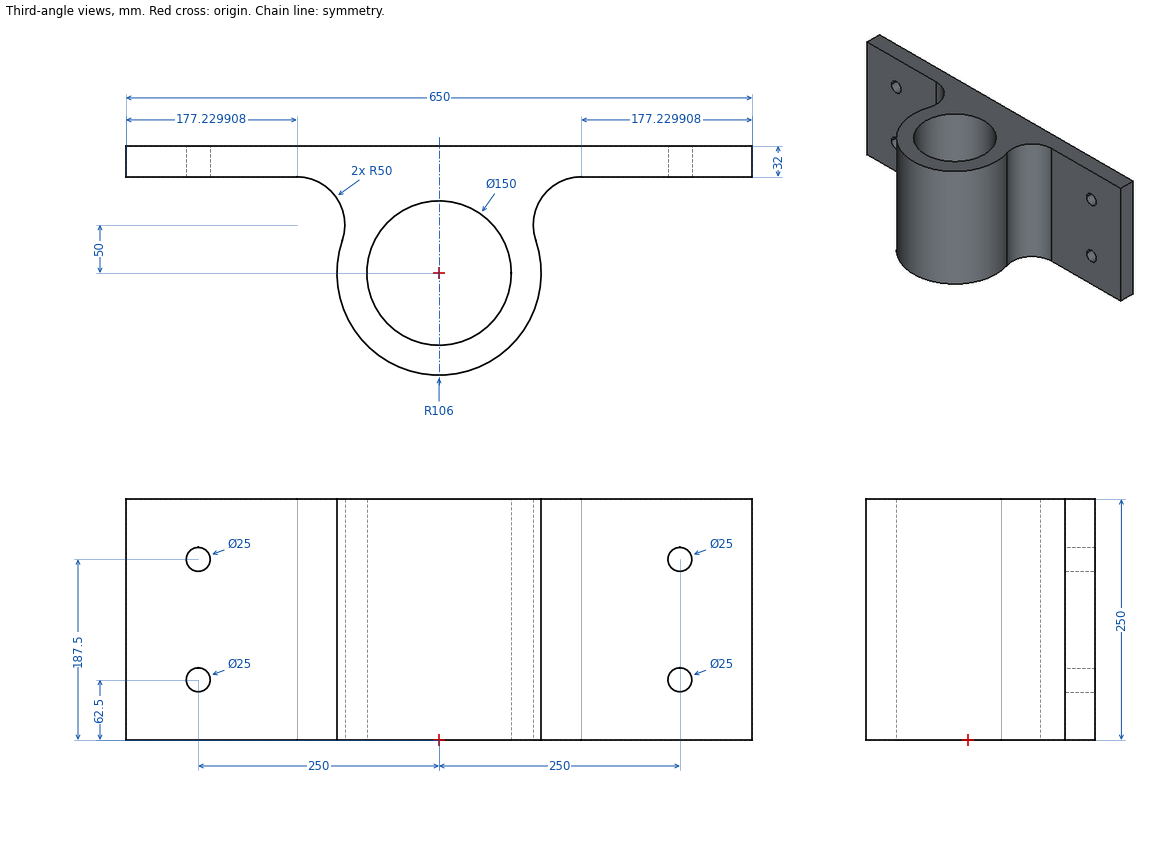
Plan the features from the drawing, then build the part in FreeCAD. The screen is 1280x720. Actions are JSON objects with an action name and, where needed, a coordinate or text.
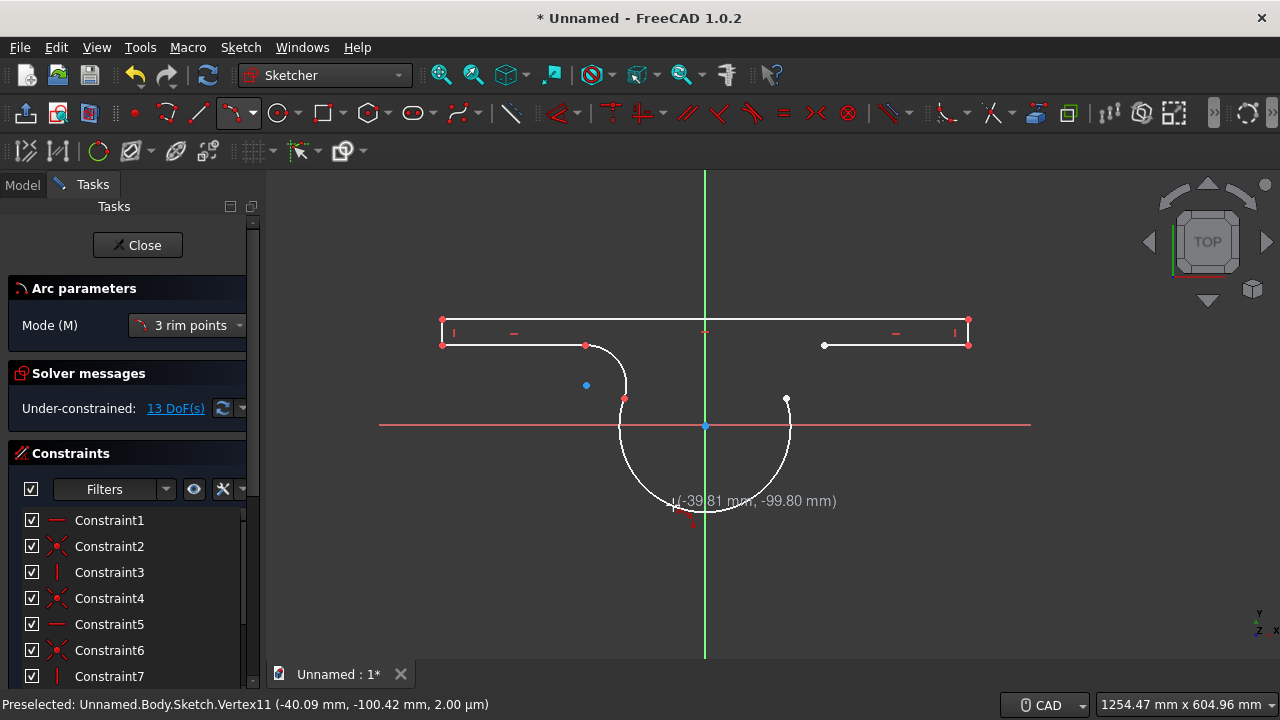
{"action": "left_click", "coordinate": [786, 399]}
{"action": "left_click", "coordinate": [825, 345]}
{"action": "left_click", "coordinate": [792, 361]}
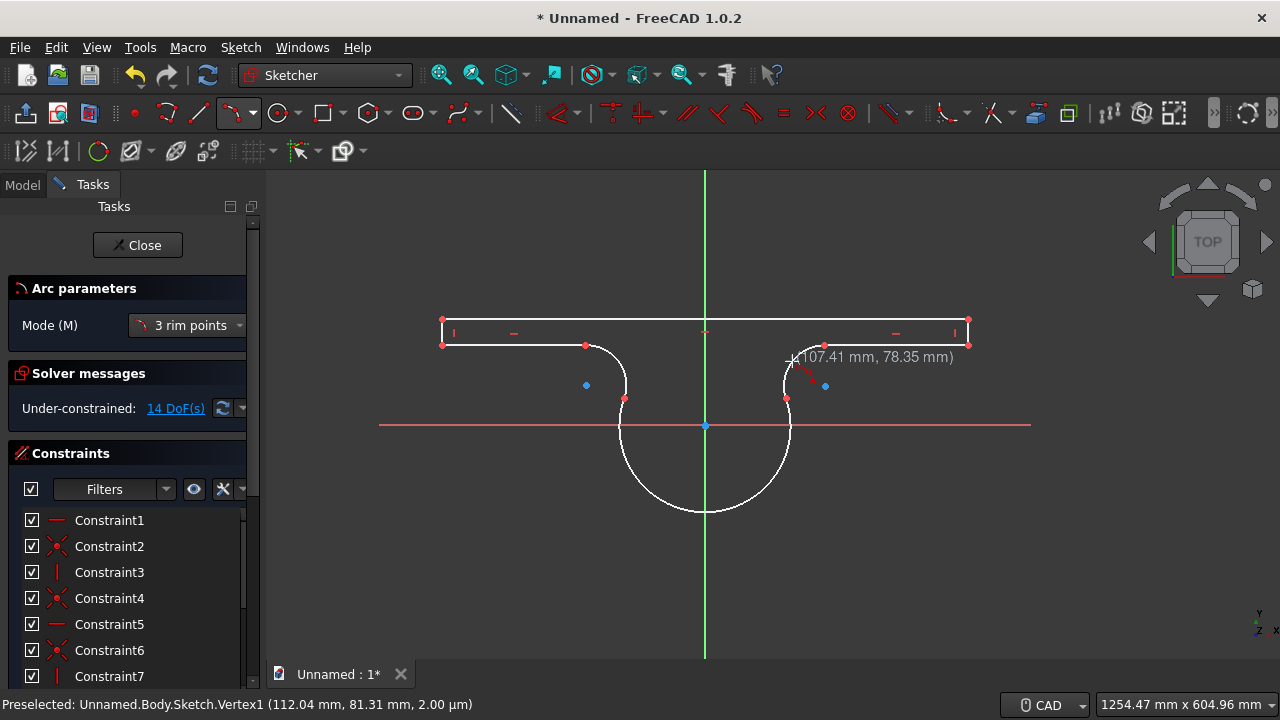
{"action": "left_click", "coordinate": [278, 114]}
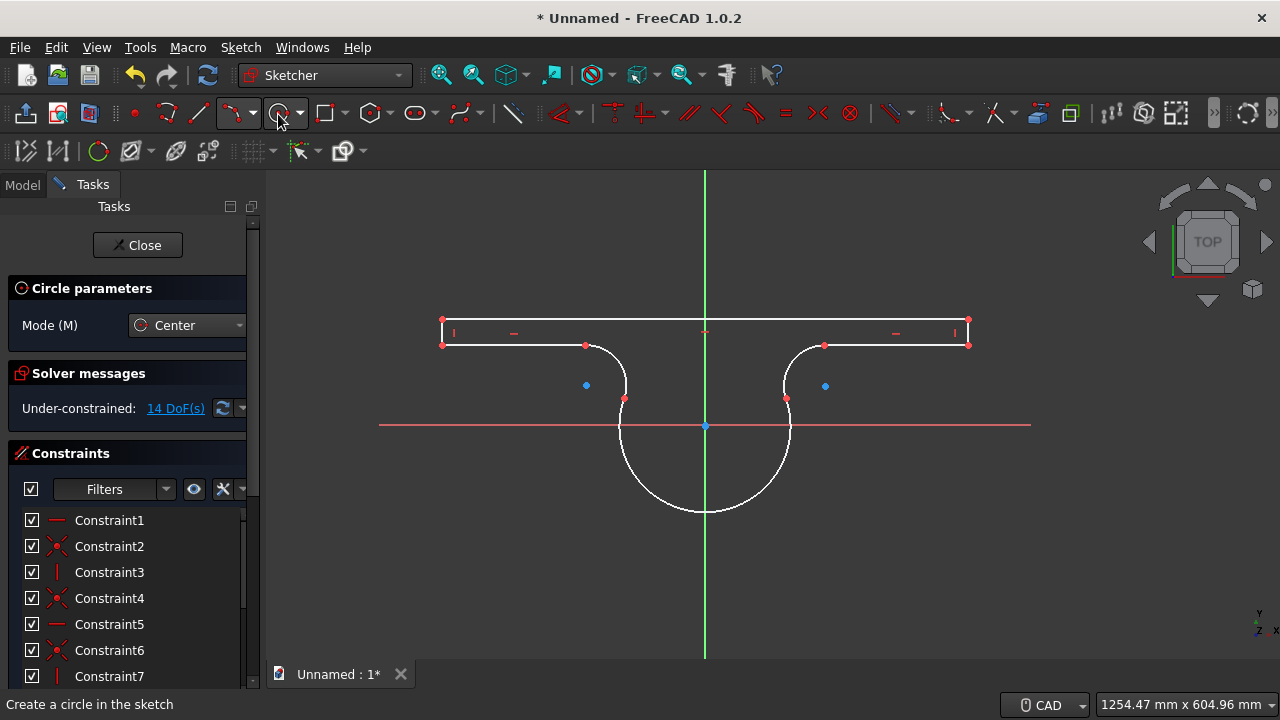
{"action": "left_click", "coordinate": [705, 425]}
{"action": "mouse_move", "coordinate": [748, 382]}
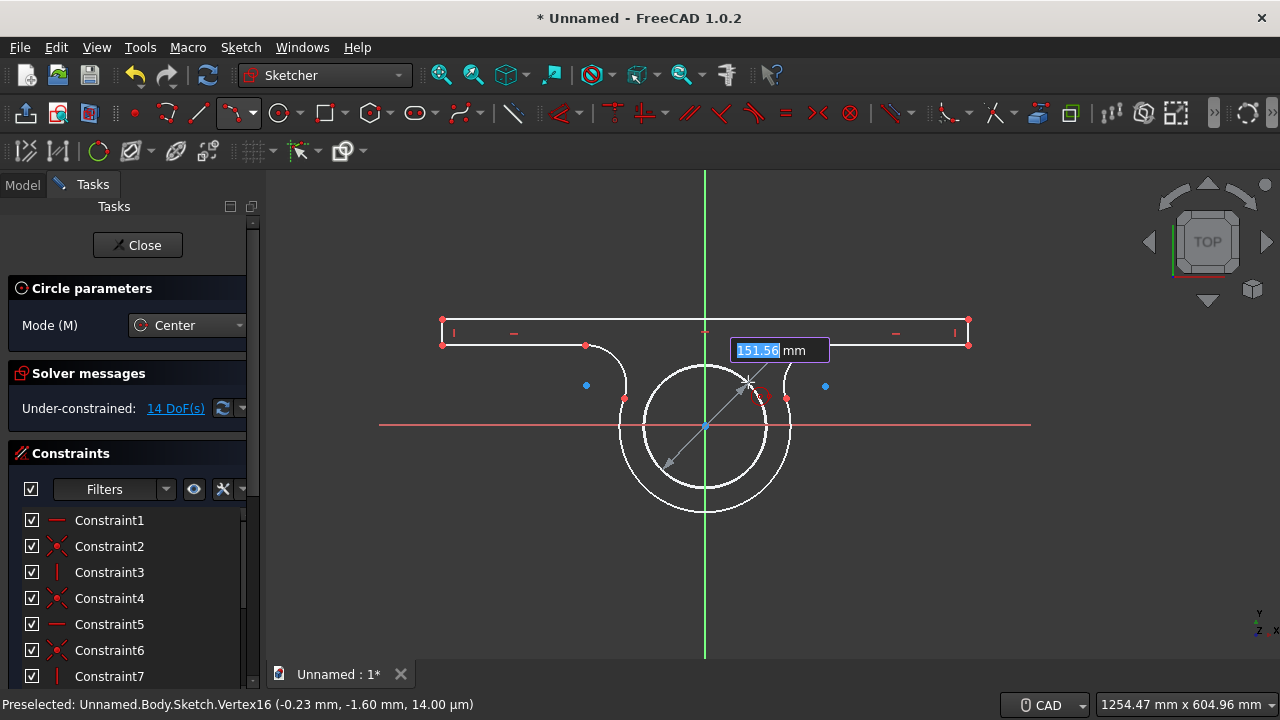
{"action": "type", "text": "150"}
{"action": "key", "text": "Return"}
{"action": "key", "text": "Escape"}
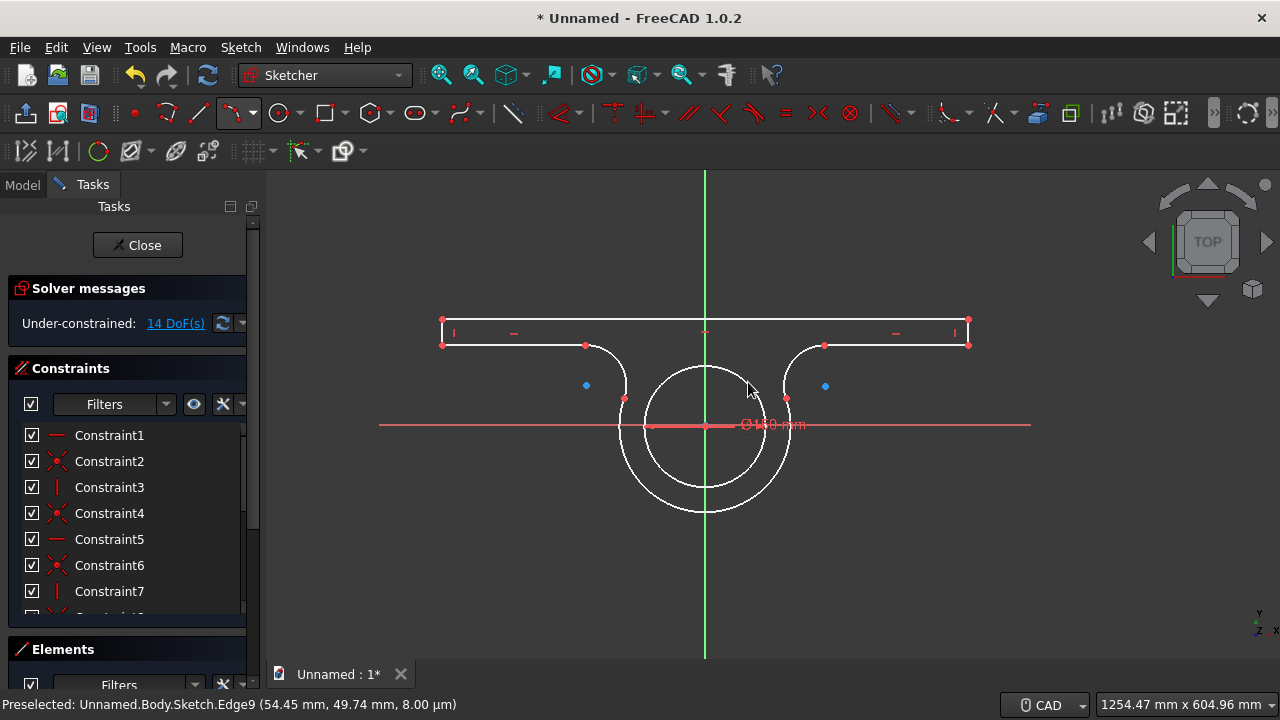
{"action": "left_click", "coordinate": [625, 376]}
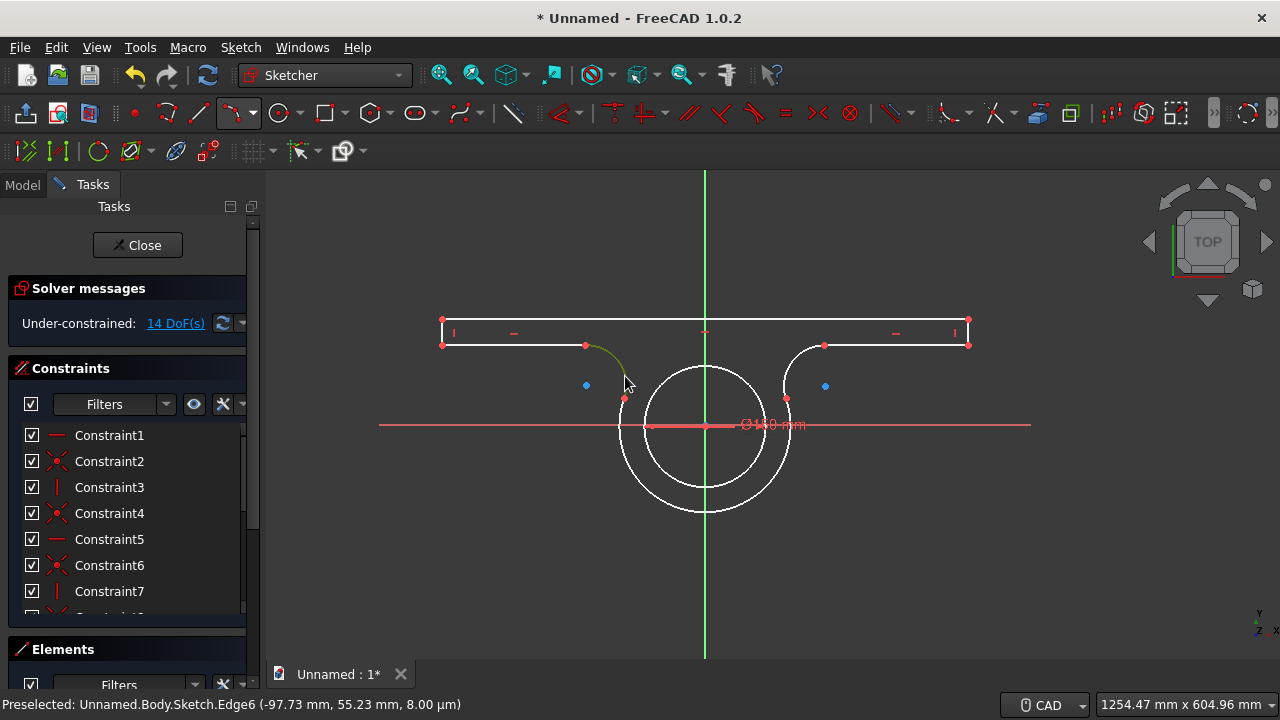
{"action": "left_click", "coordinate": [646, 489]}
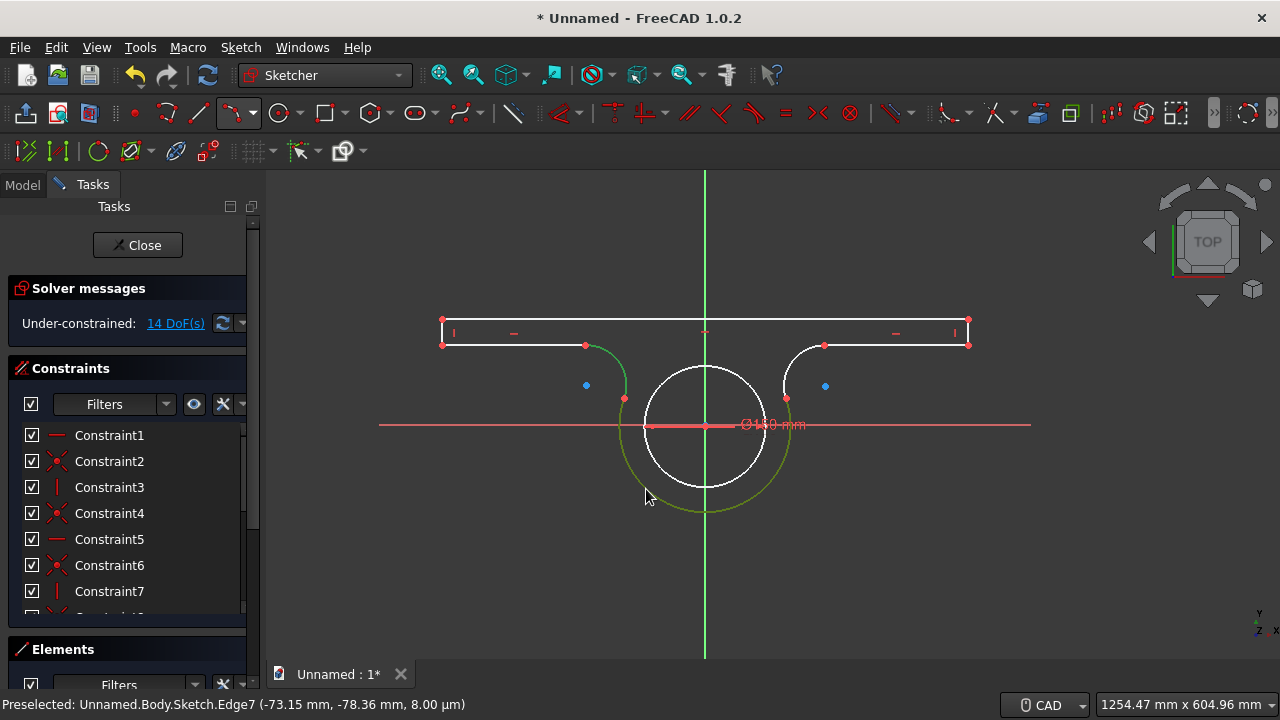
{"action": "left_click", "coordinate": [754, 114]}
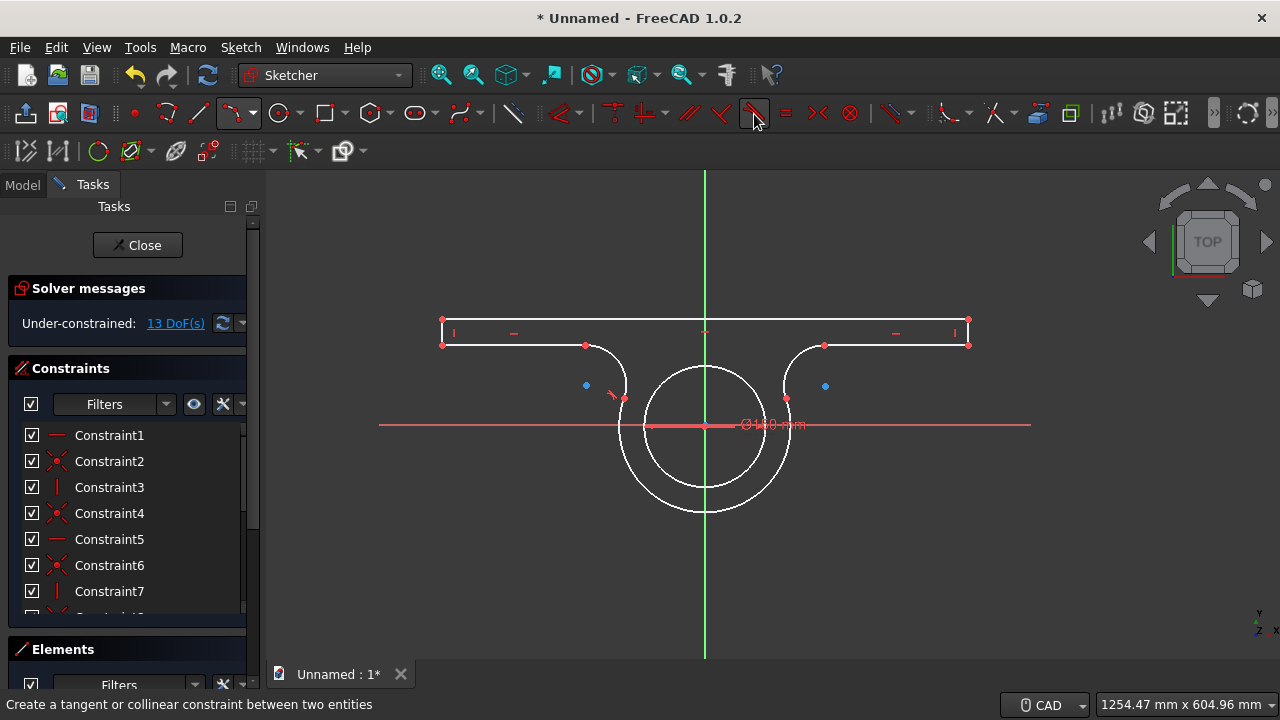
{"action": "left_click", "coordinate": [645, 488]}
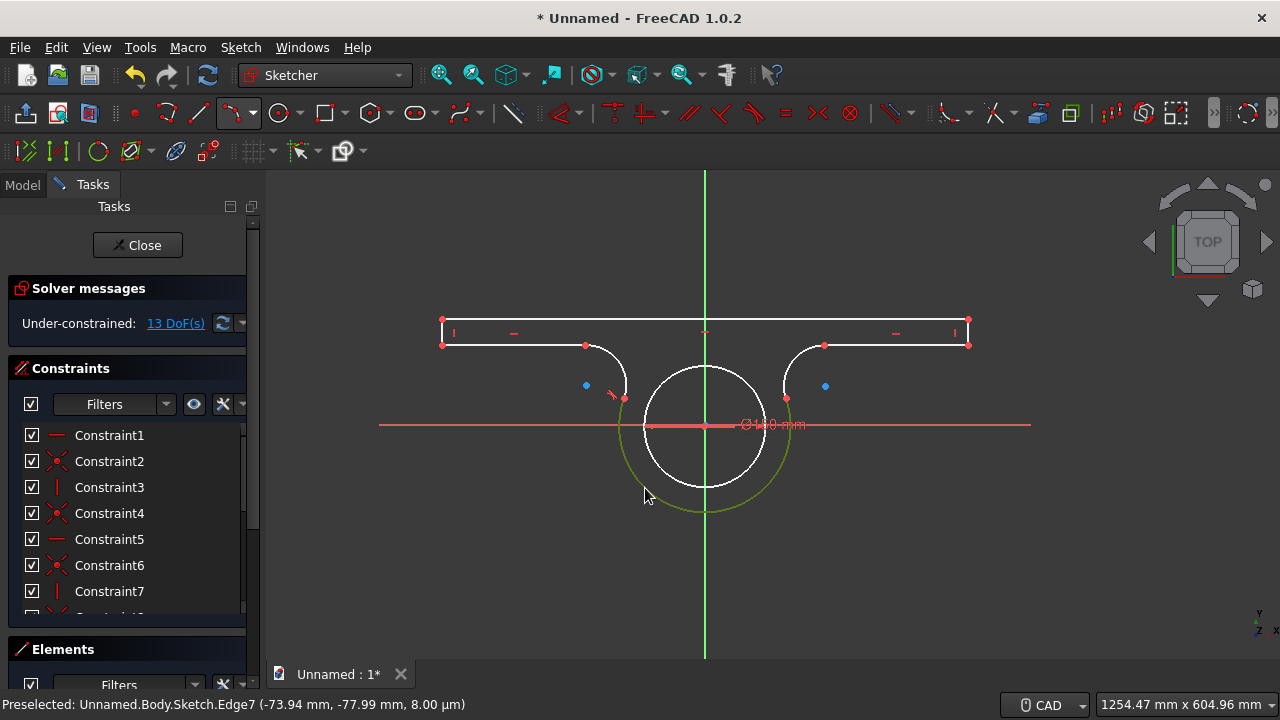
{"action": "left_click", "coordinate": [803, 352]}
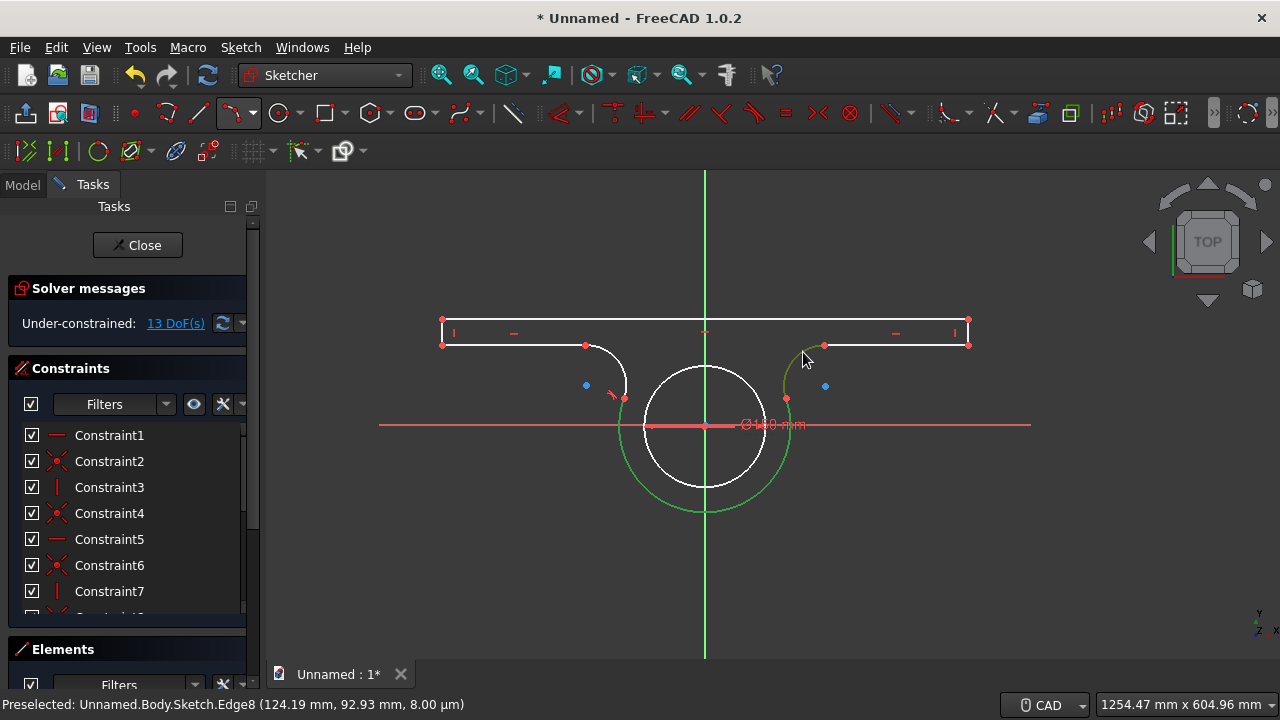
{"action": "key", "text": "t"}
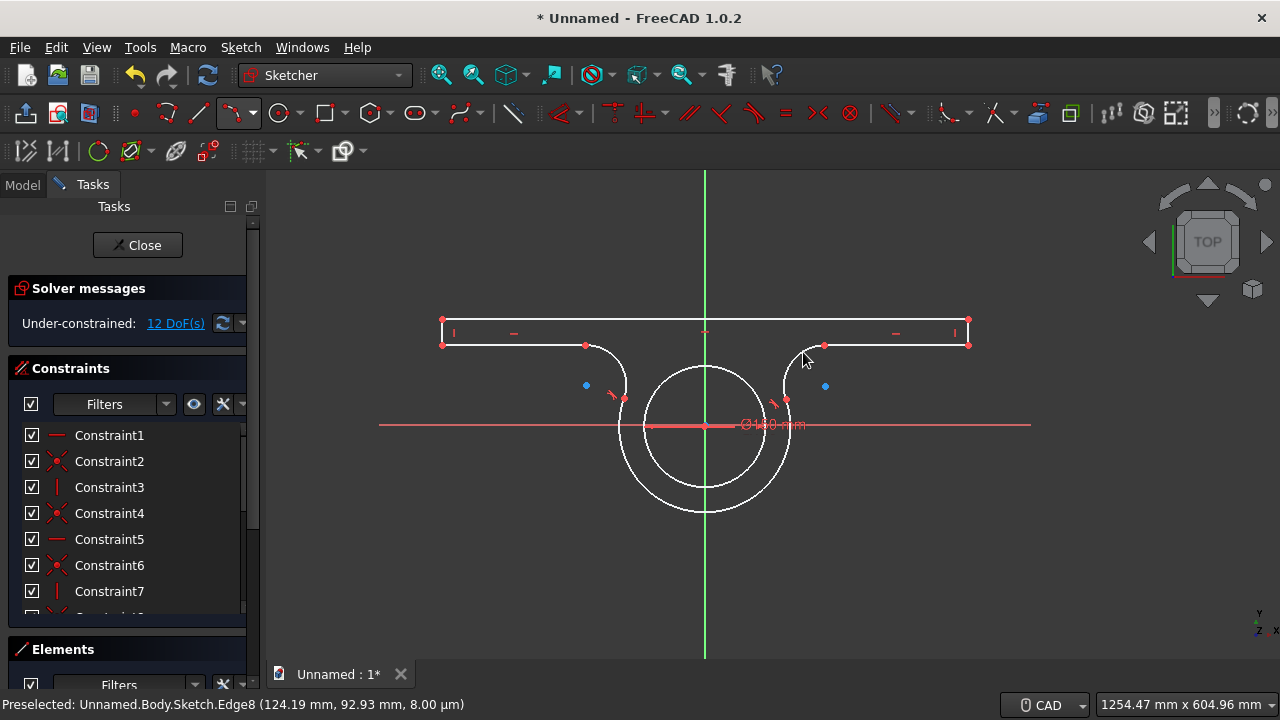
{"action": "left_click_drag", "start_coordinate": [695, 415], "coordinate": [715, 437]}